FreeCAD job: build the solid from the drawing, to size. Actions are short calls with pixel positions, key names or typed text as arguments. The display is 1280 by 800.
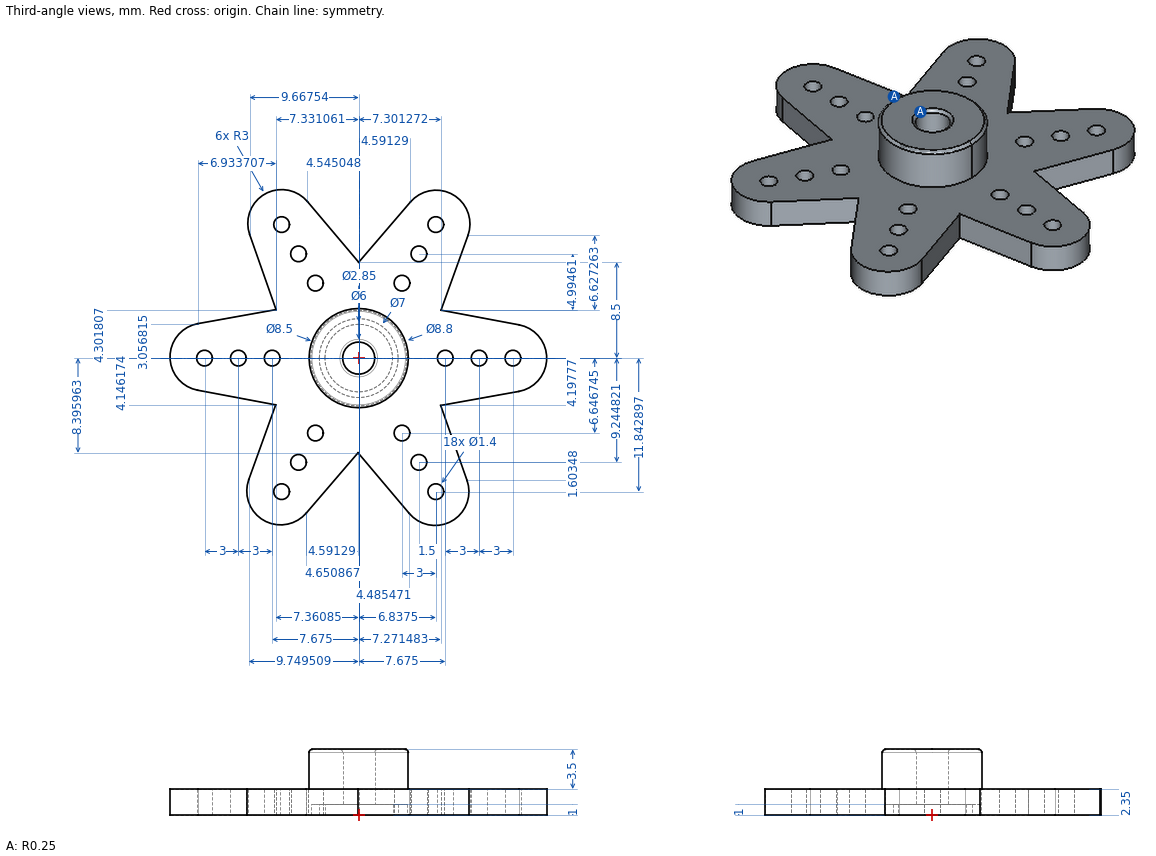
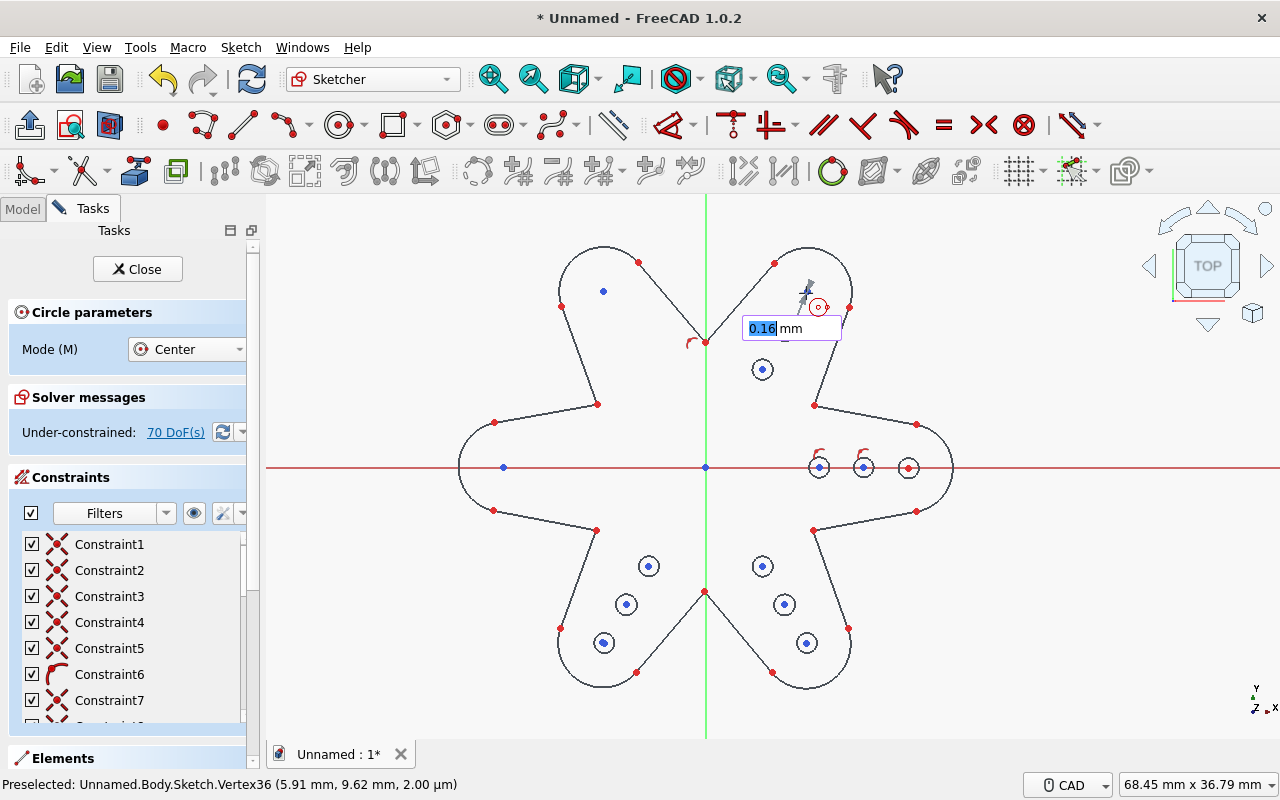
scroll(814, 285, up, 3)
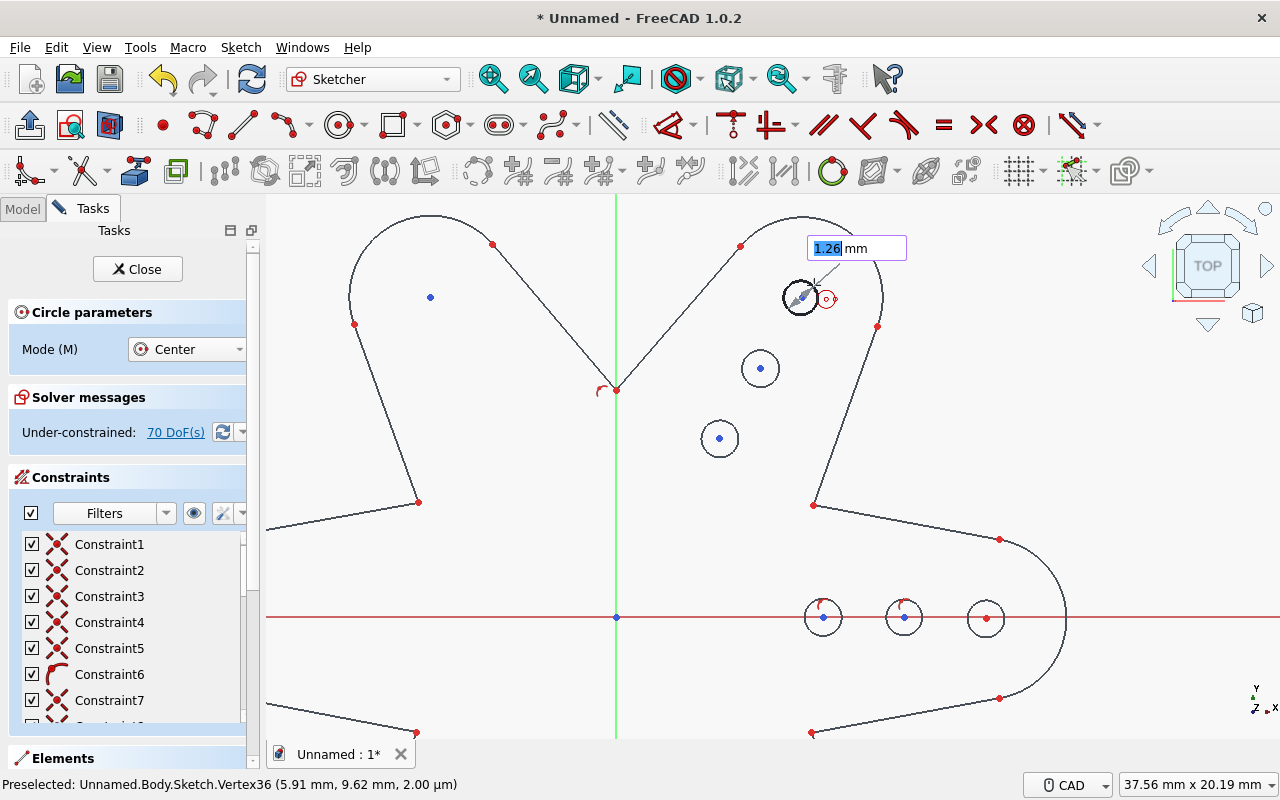
click(814, 284)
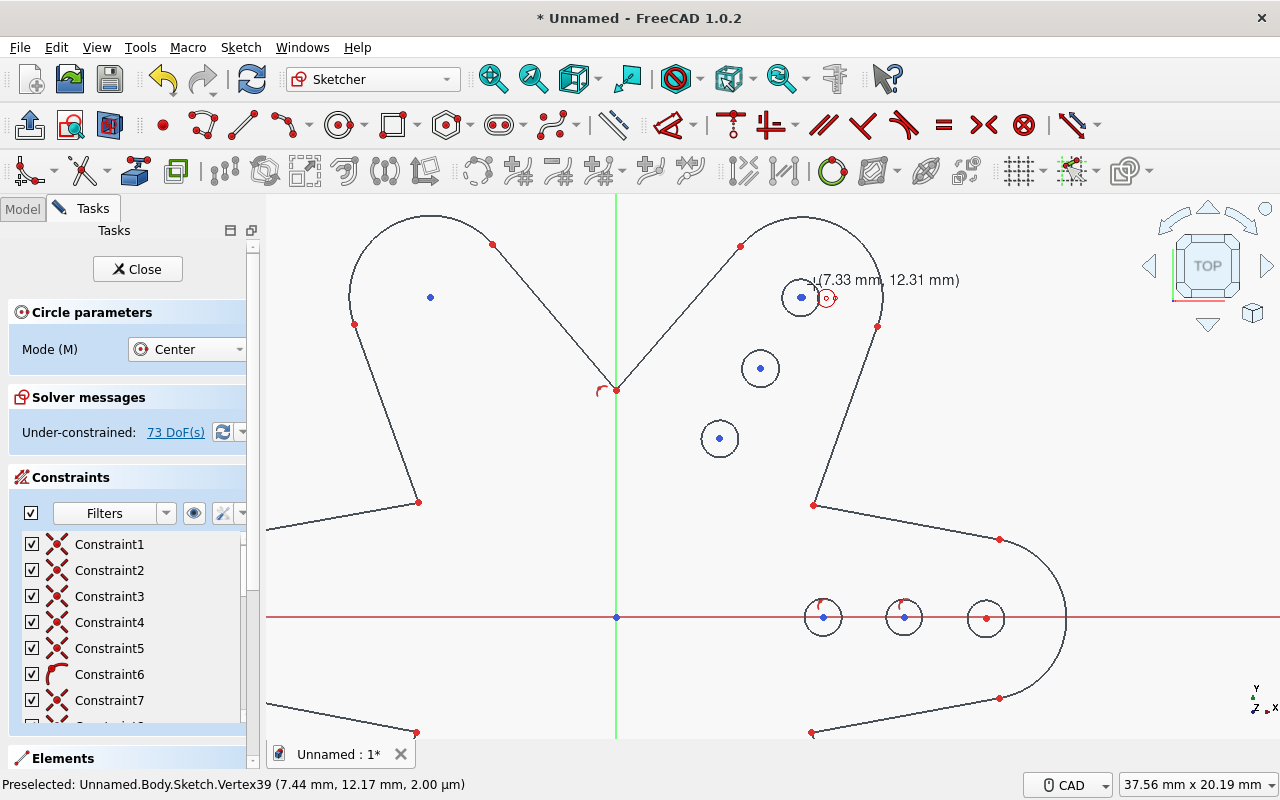
click(409, 617)
click(415, 600)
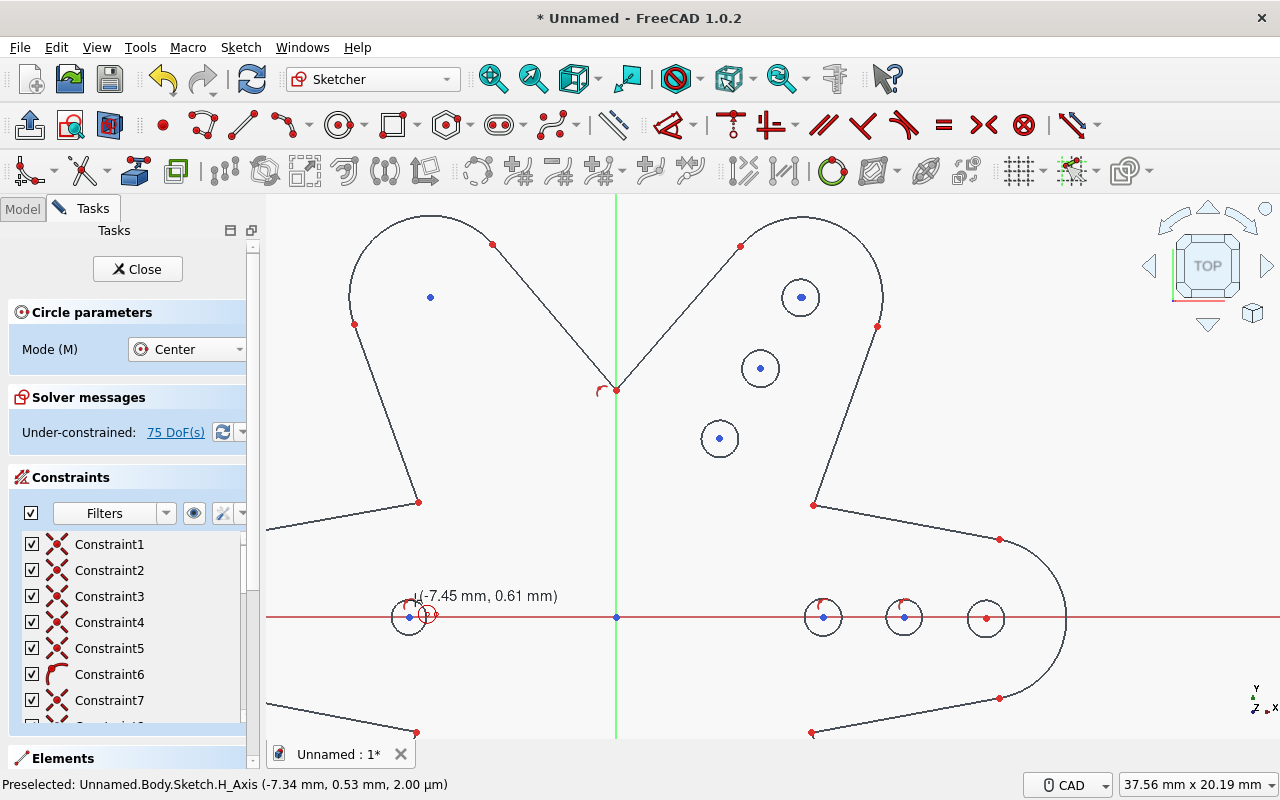
click(328, 617)
click(334, 600)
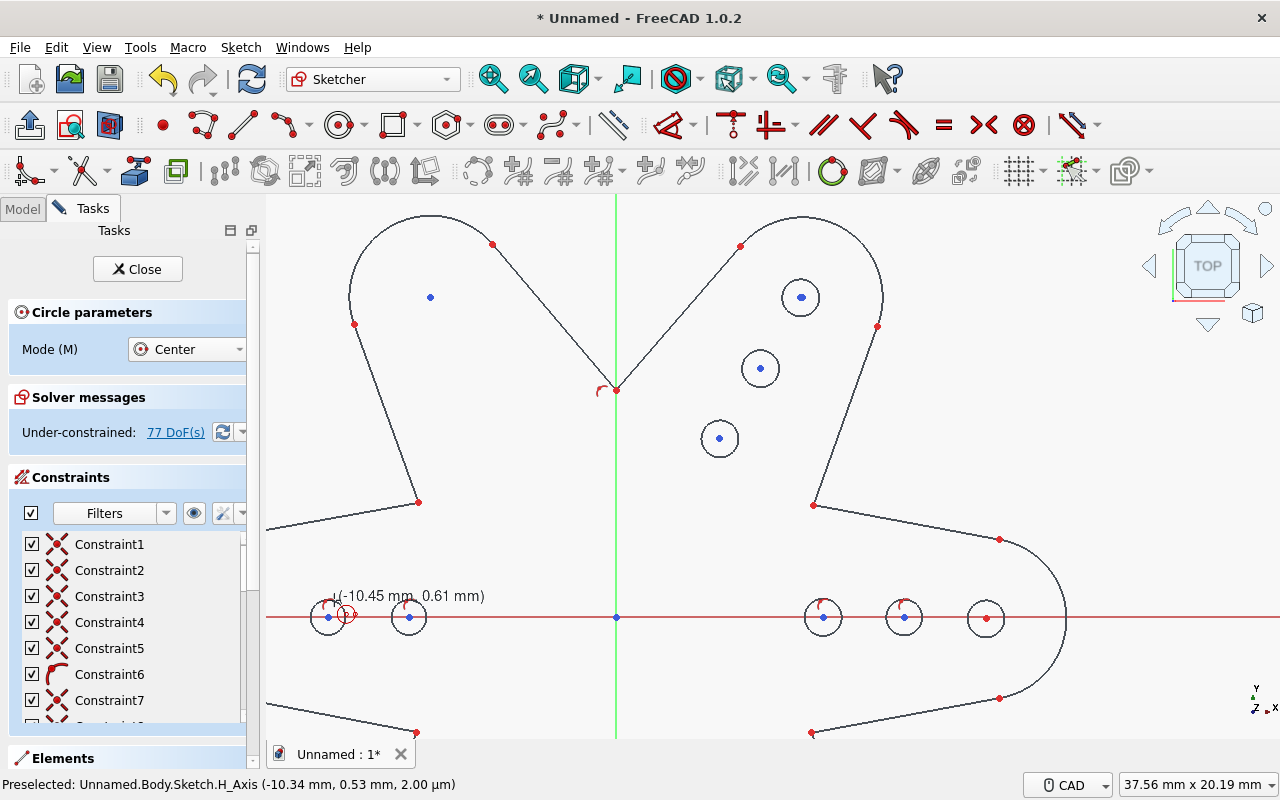
scroll(777, 345, down, 4)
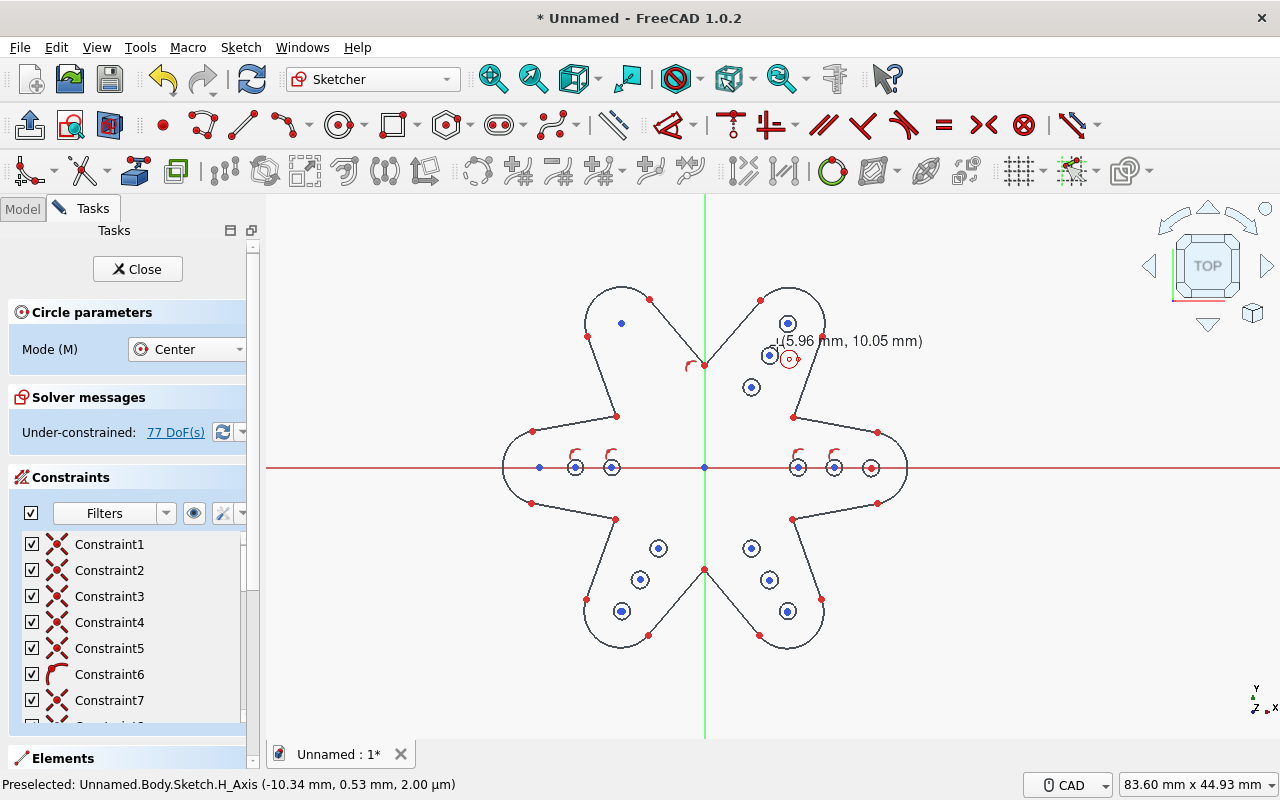
scroll(539, 468, up, 12)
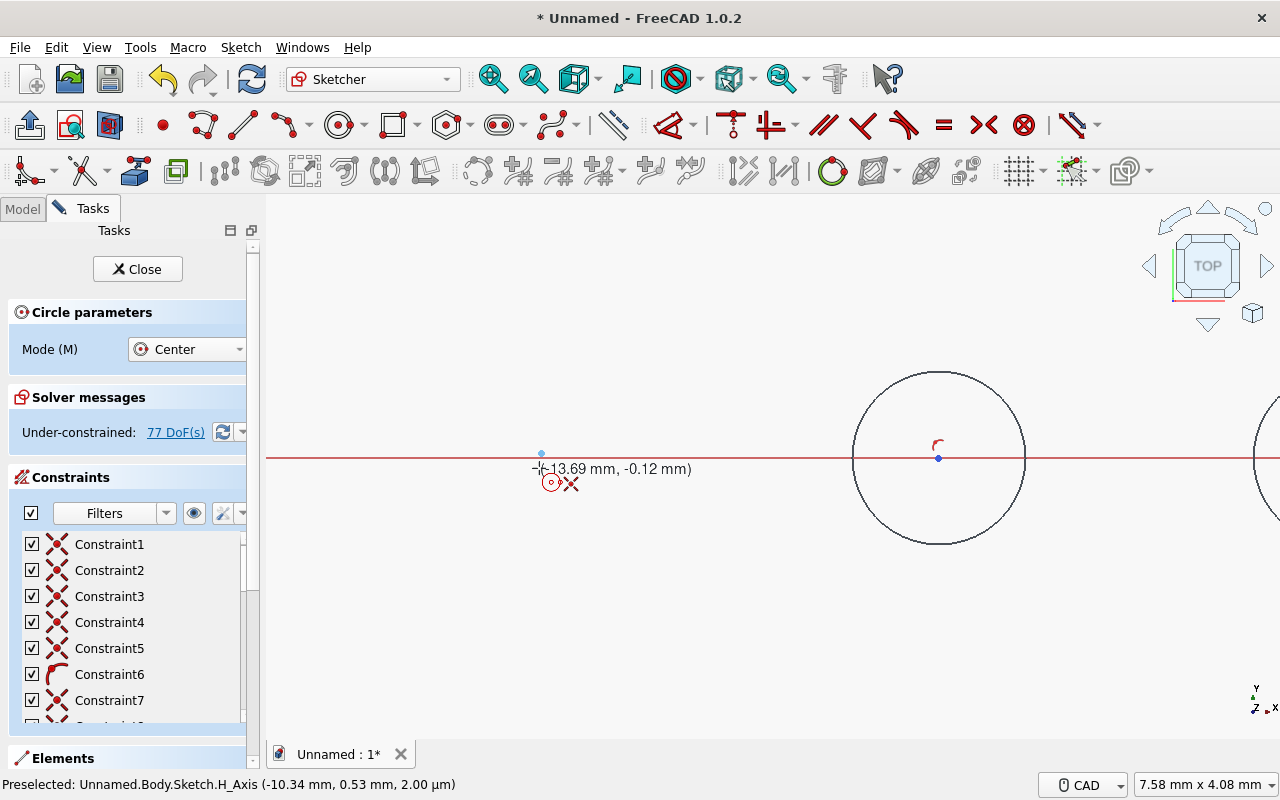
click(538, 458)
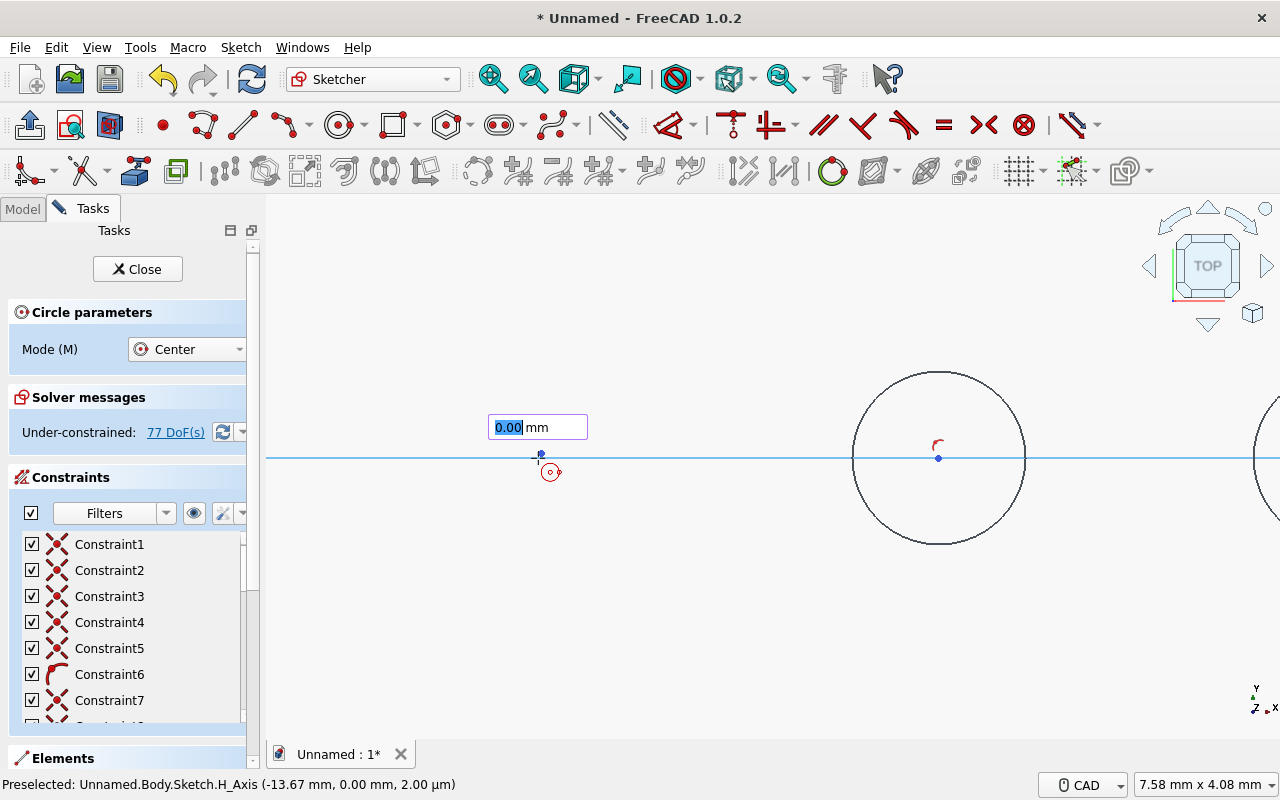
scroll(539, 468, down, 12)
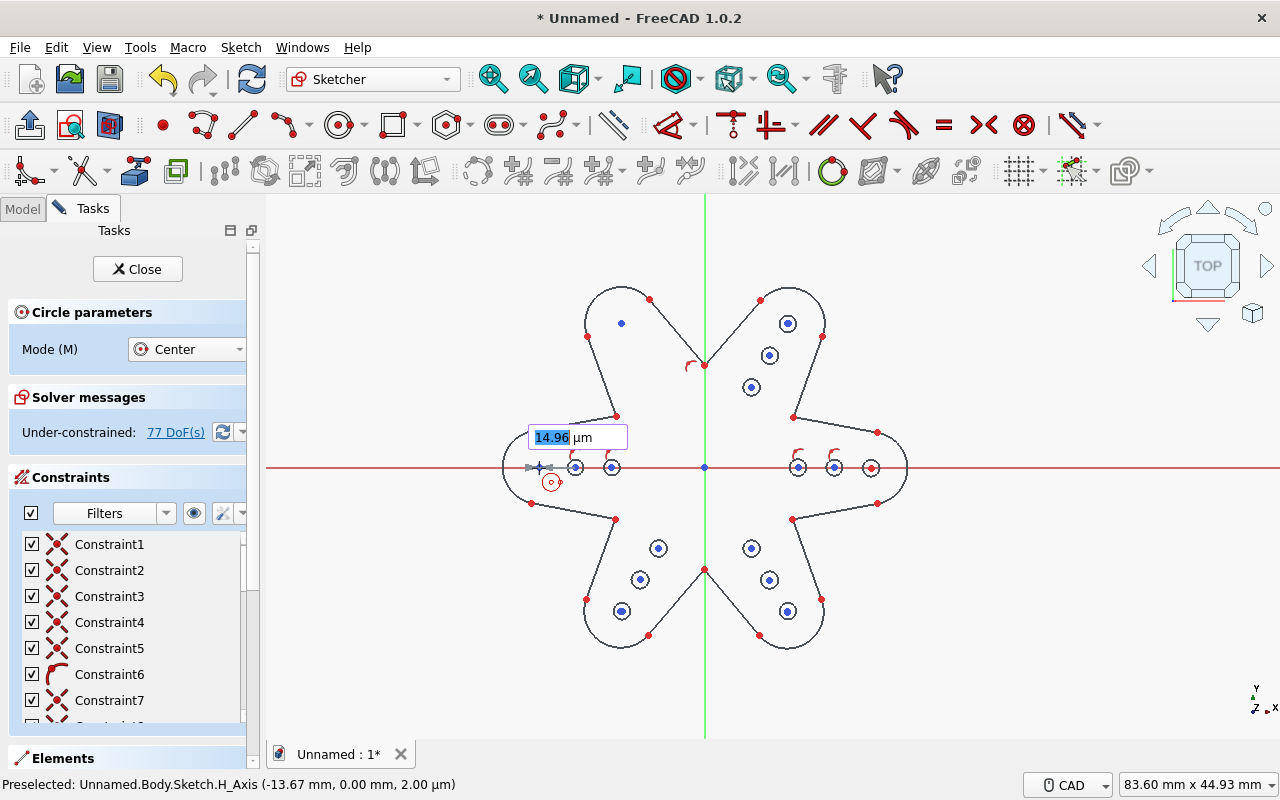
scroll(545, 462, up, 5)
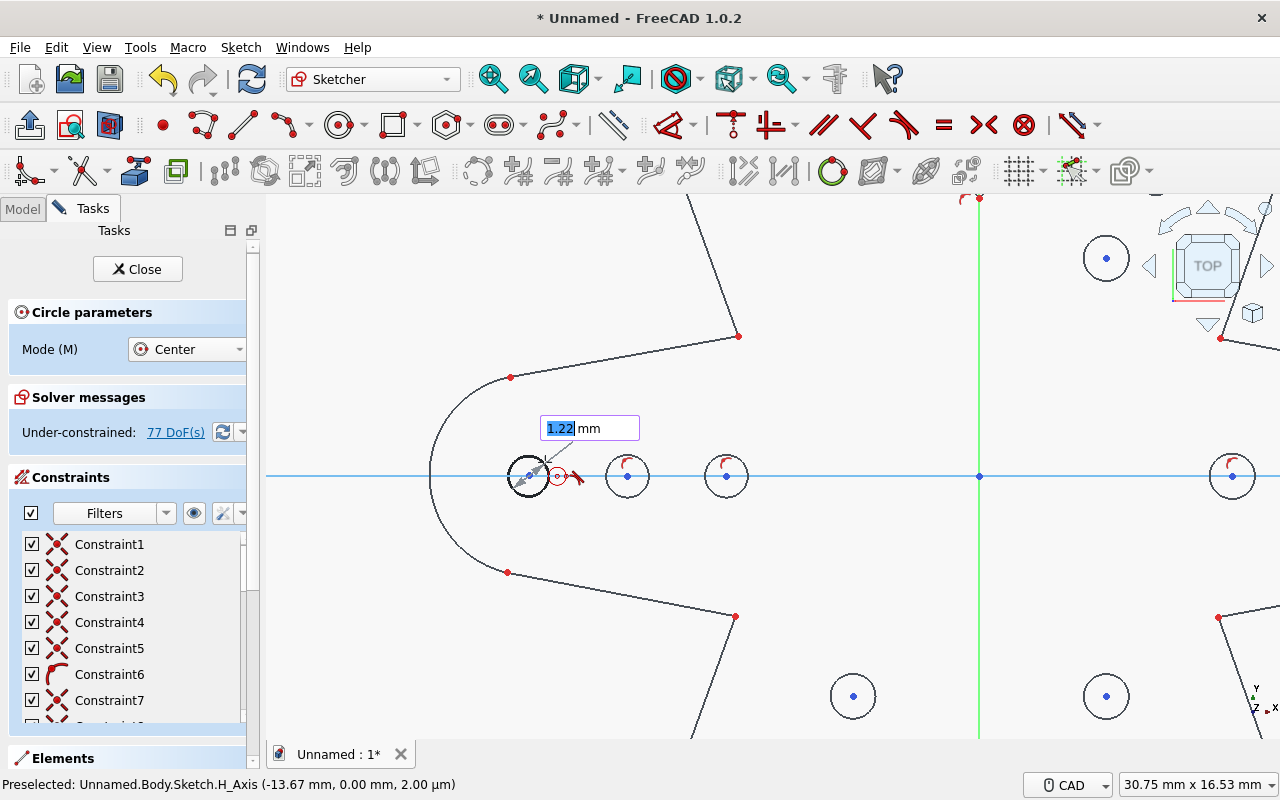
click(545, 460)